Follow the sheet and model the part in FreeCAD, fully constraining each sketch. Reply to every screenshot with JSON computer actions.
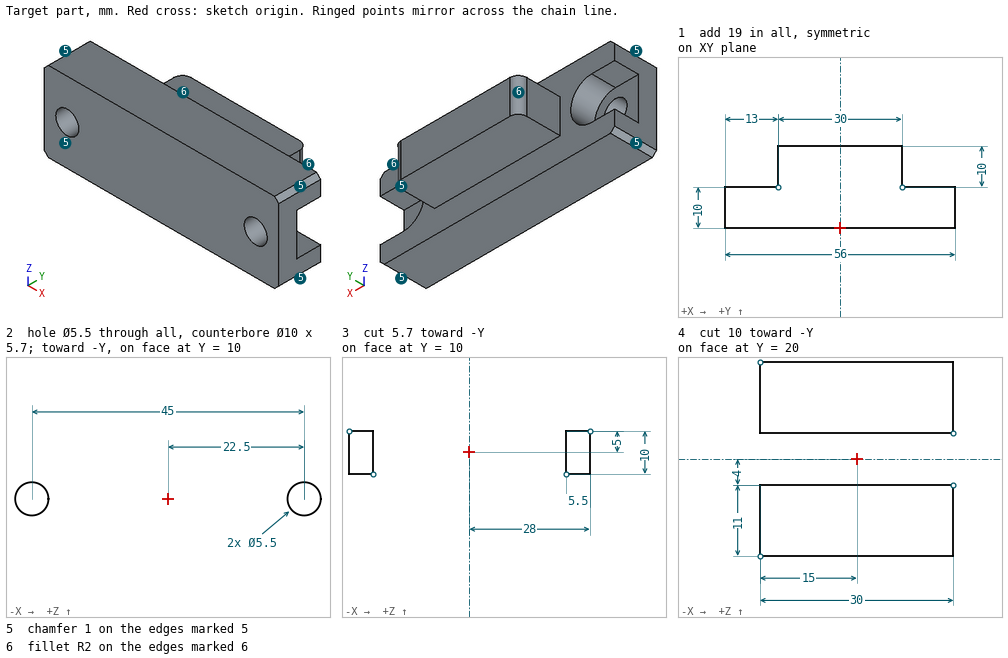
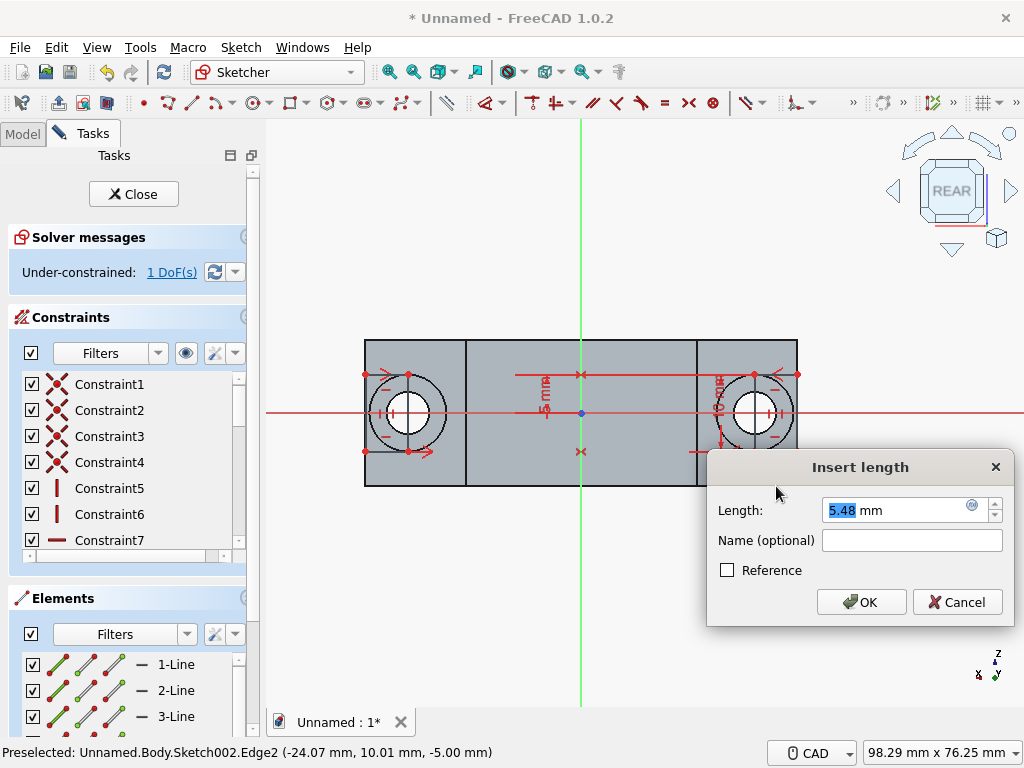
{"action": "type", "text": "5.5"}
{"action": "key", "text": "Return"}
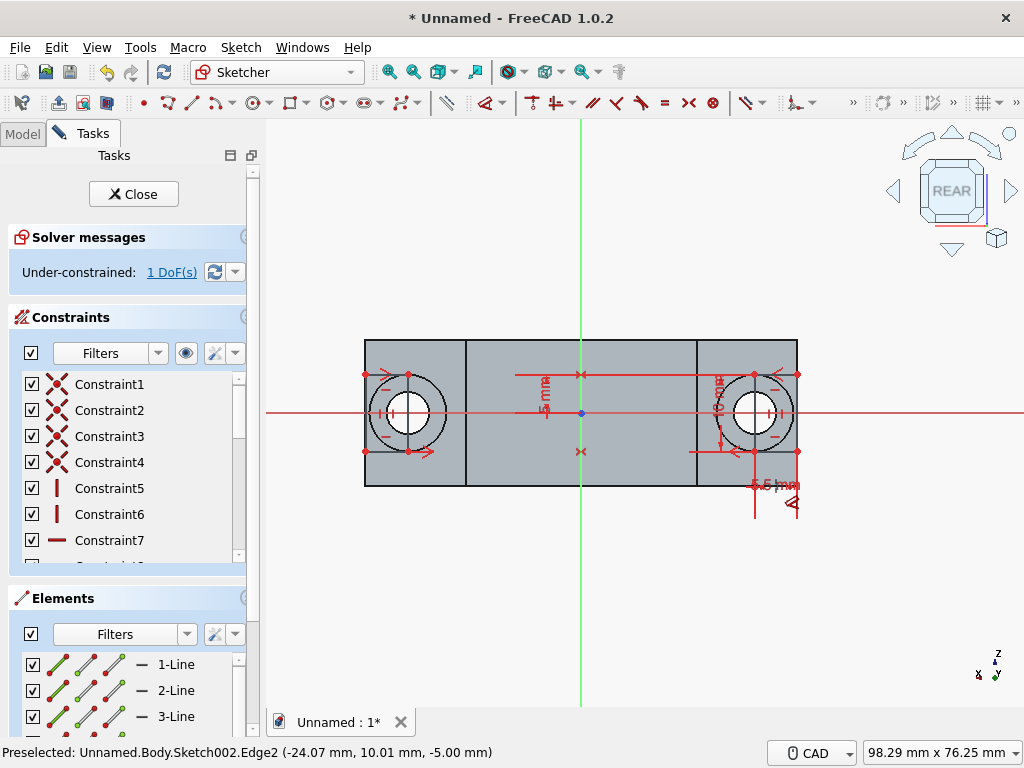
{"action": "left_click", "coordinate": [797, 452]}
{"action": "left_click", "coordinate": [689, 486]}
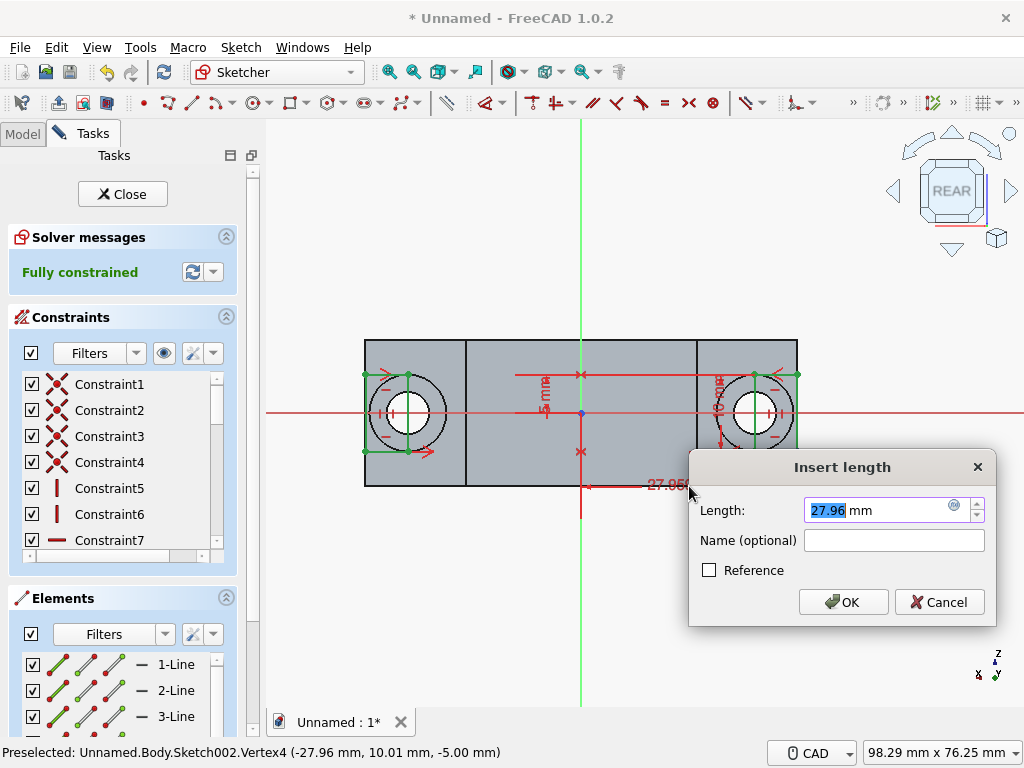
{"action": "type", "text": "28"}
{"action": "key", "text": "Return"}
{"action": "key", "text": "Escape"}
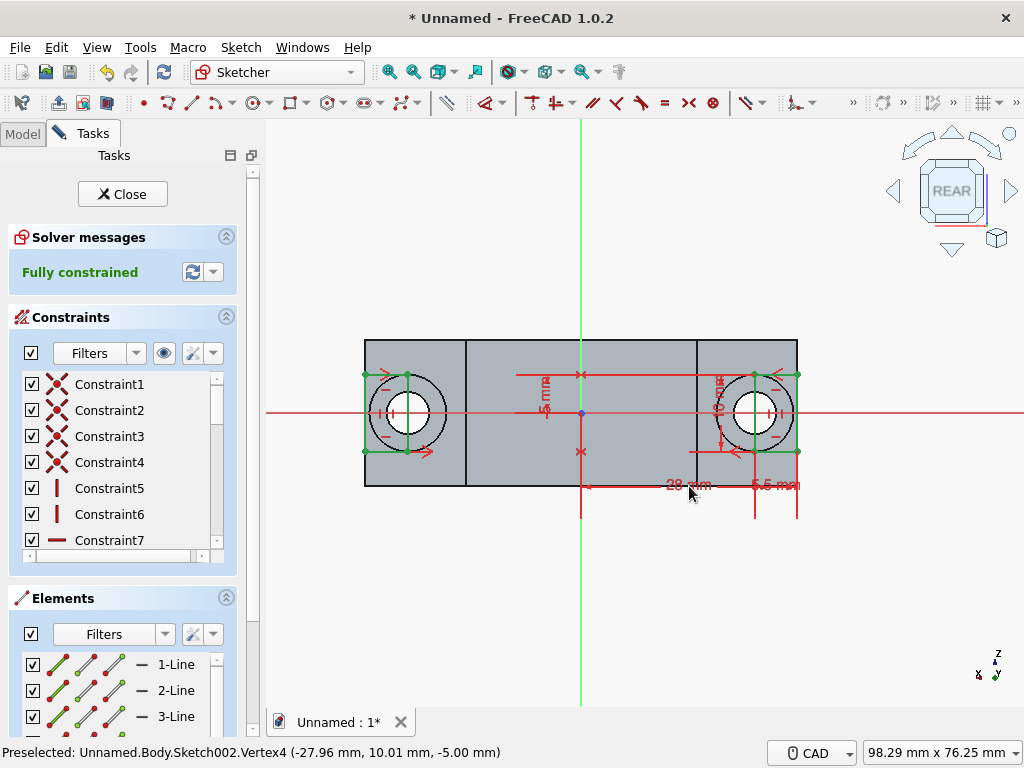
{"action": "left_click", "coordinate": [123, 194]}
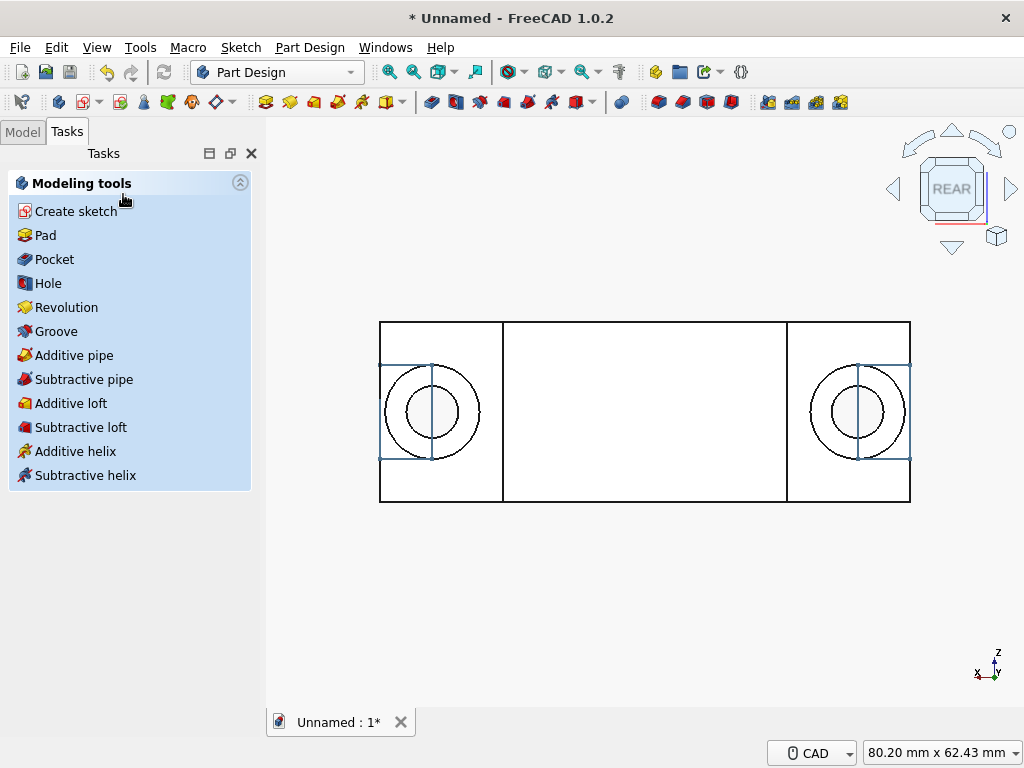
{"action": "left_click", "coordinate": [432, 102]}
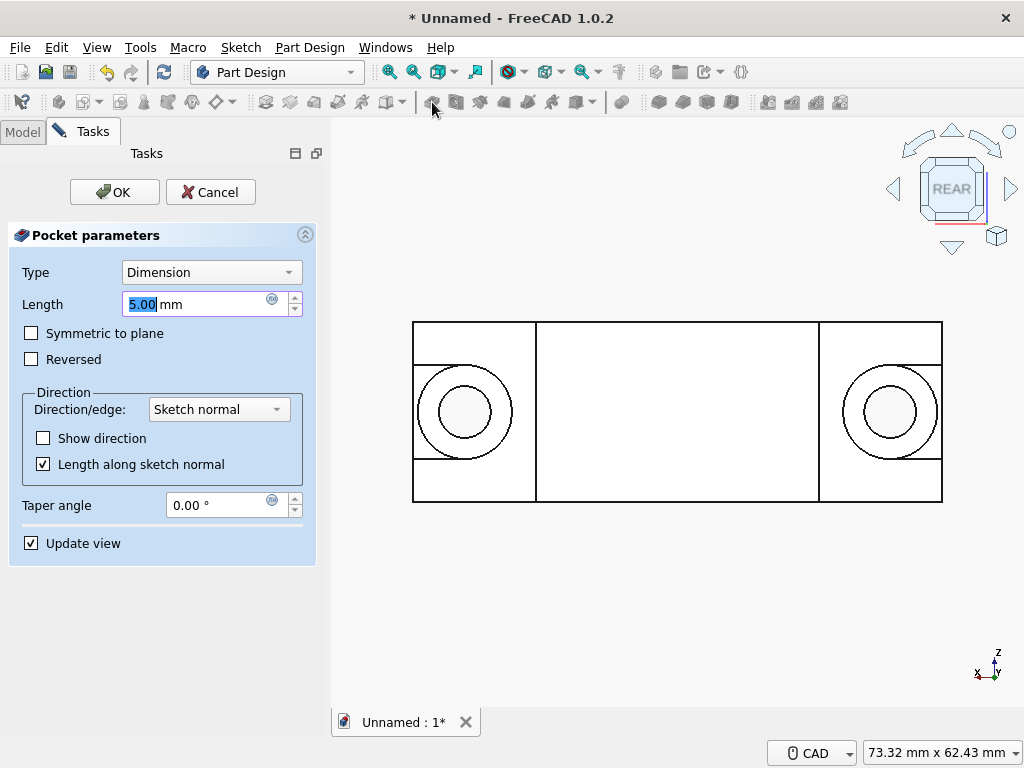
{"action": "type", "text": "5.7"}
{"action": "key", "text": "Tab"}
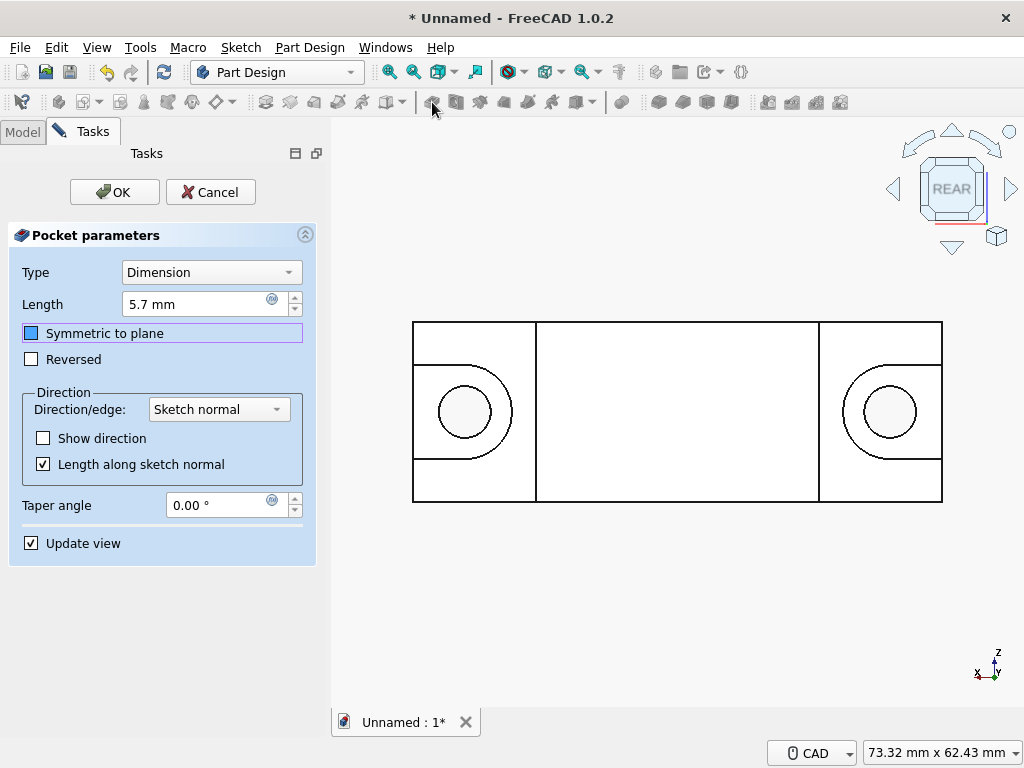
{"action": "left_click", "coordinate": [115, 192]}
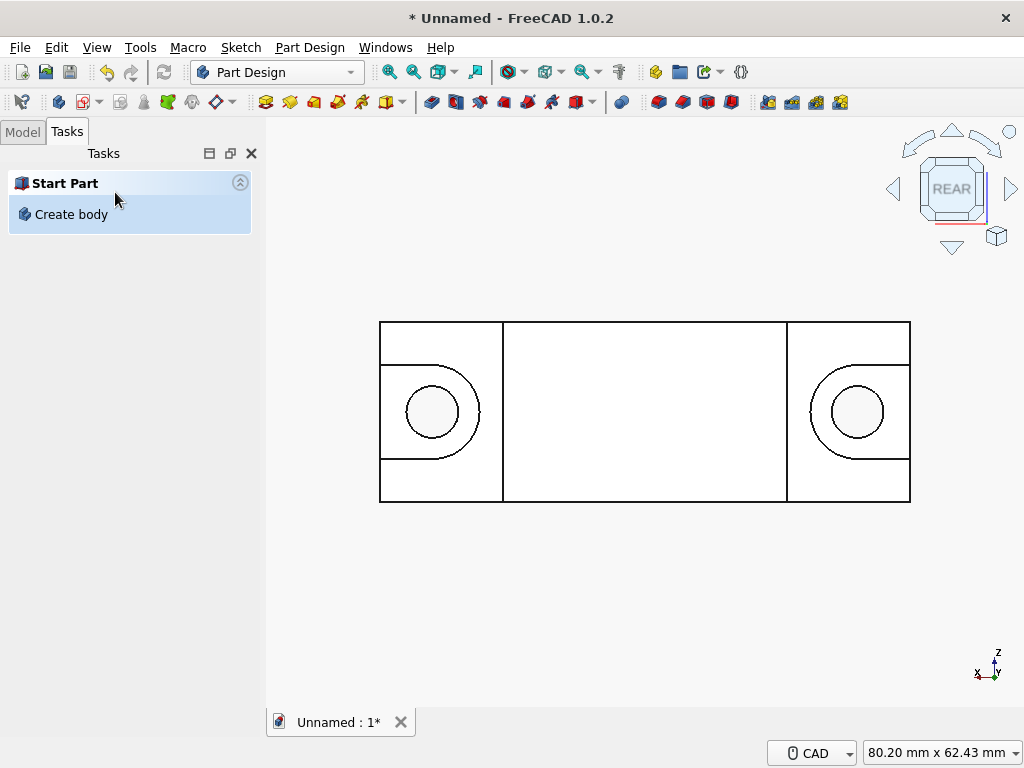
{"action": "left_click", "coordinate": [604, 411]}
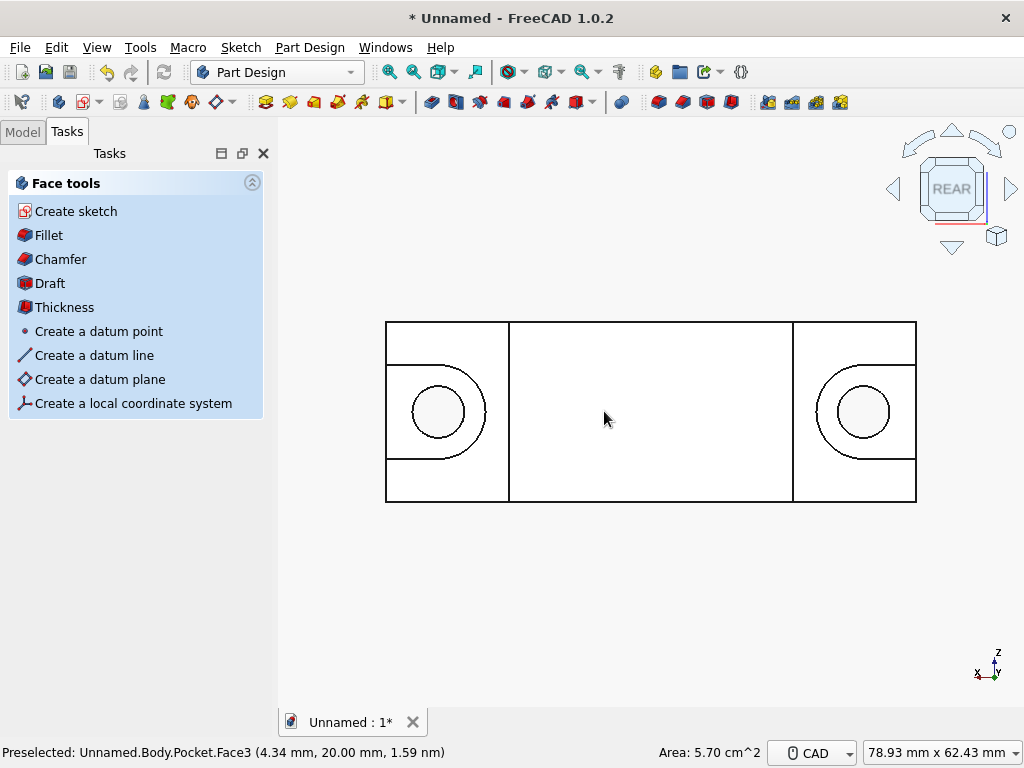
{"action": "left_click", "coordinate": [84, 102]}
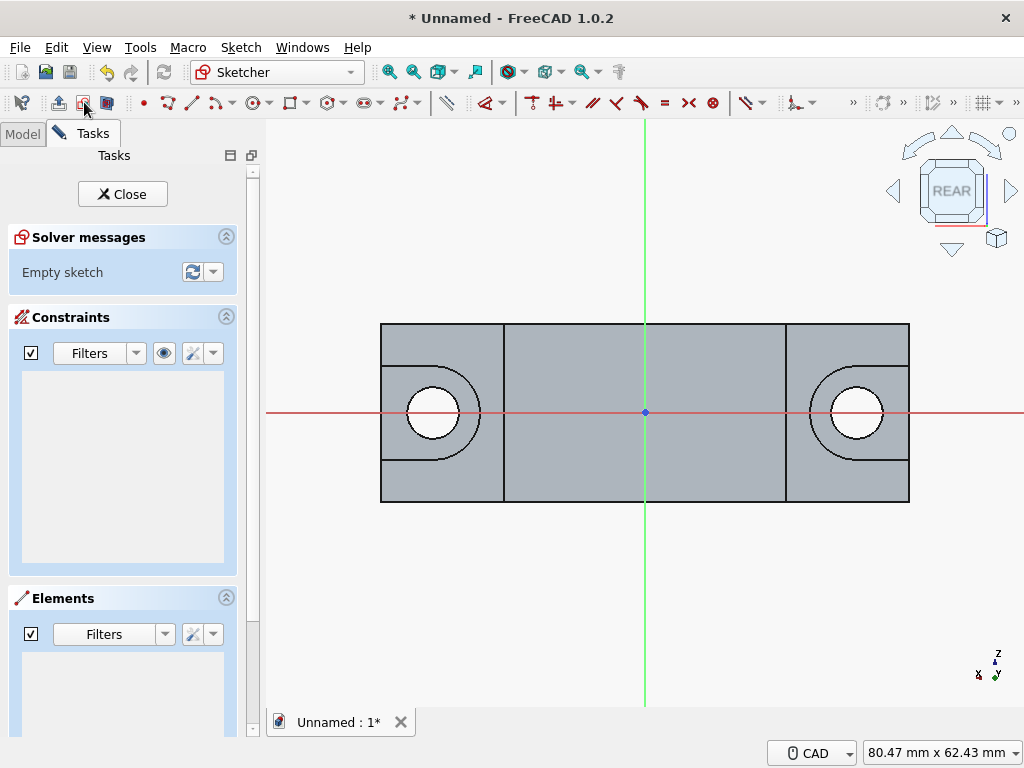
{"action": "left_click", "coordinate": [290, 104]}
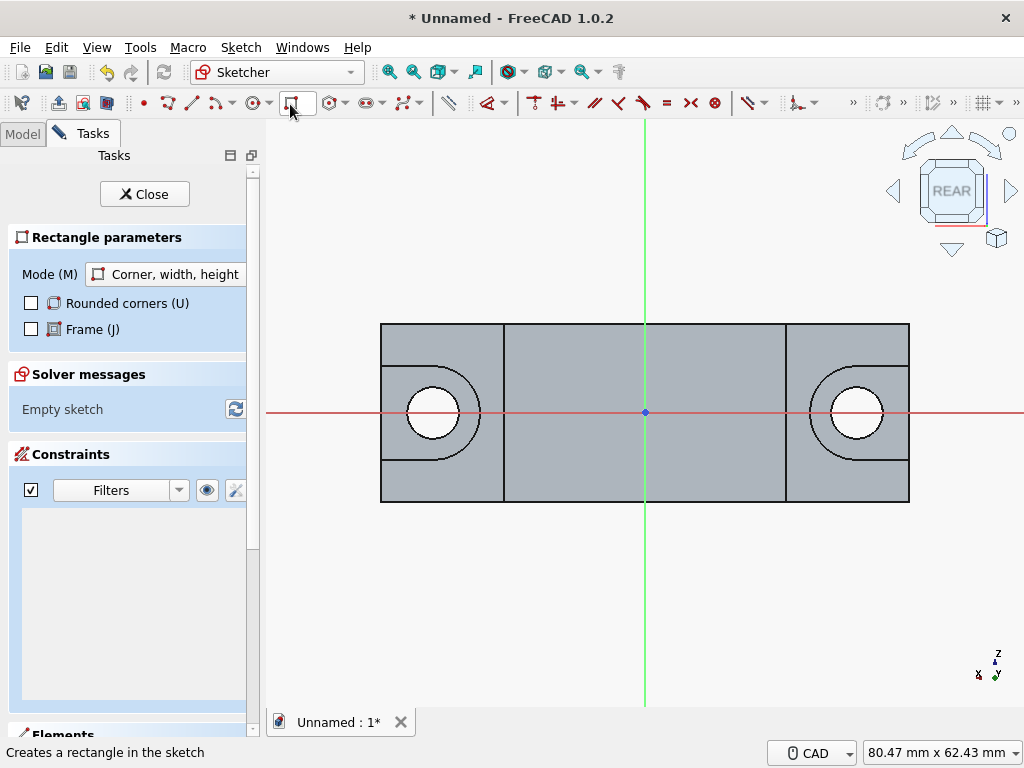
{"action": "left_click", "coordinate": [504, 451]}
{"action": "left_click", "coordinate": [786, 554]}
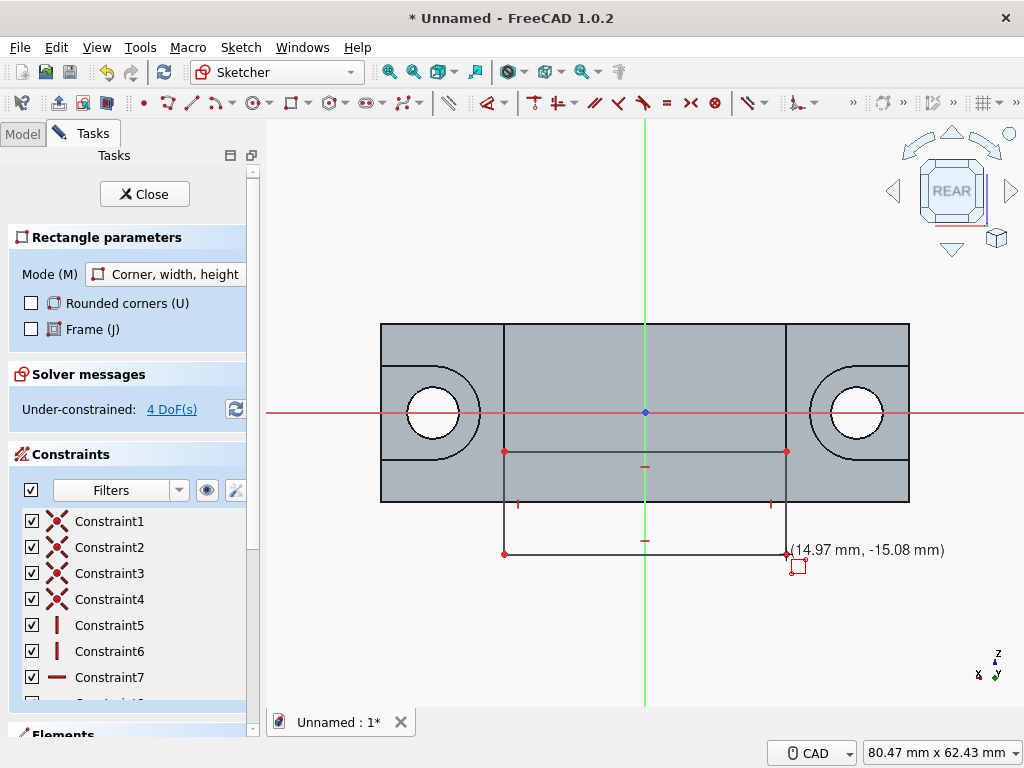
{"action": "left_click", "coordinate": [504, 272]}
{"action": "left_click", "coordinate": [786, 375]}
{"action": "key", "text": "Escape"}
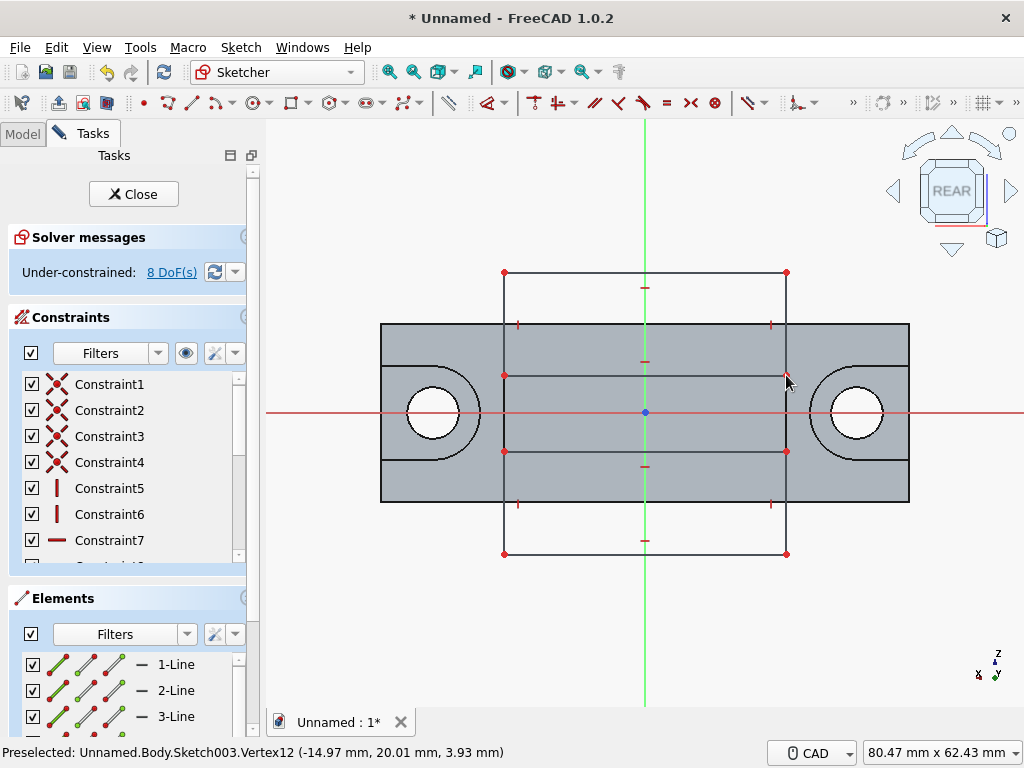
{"action": "left_click", "coordinate": [504, 555]}